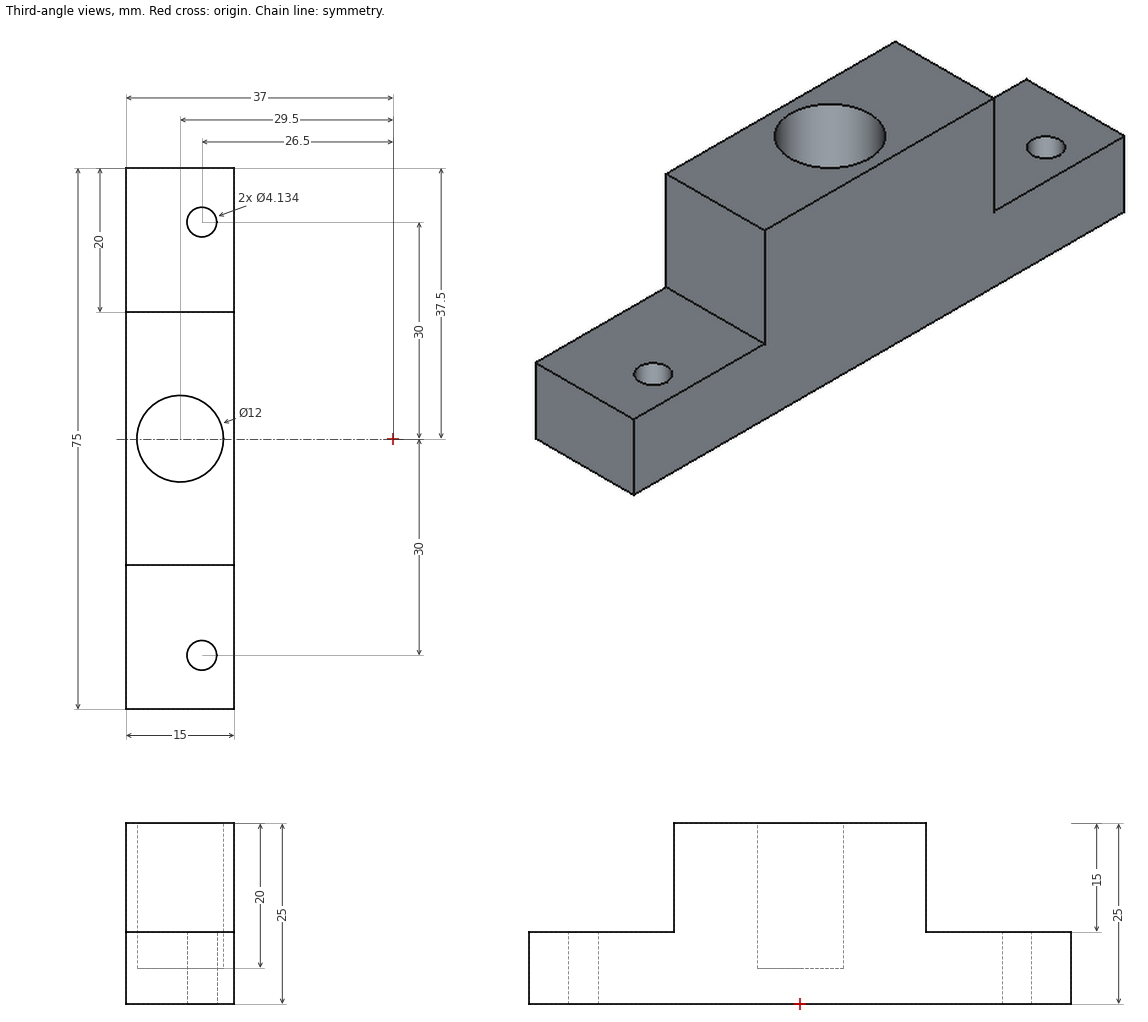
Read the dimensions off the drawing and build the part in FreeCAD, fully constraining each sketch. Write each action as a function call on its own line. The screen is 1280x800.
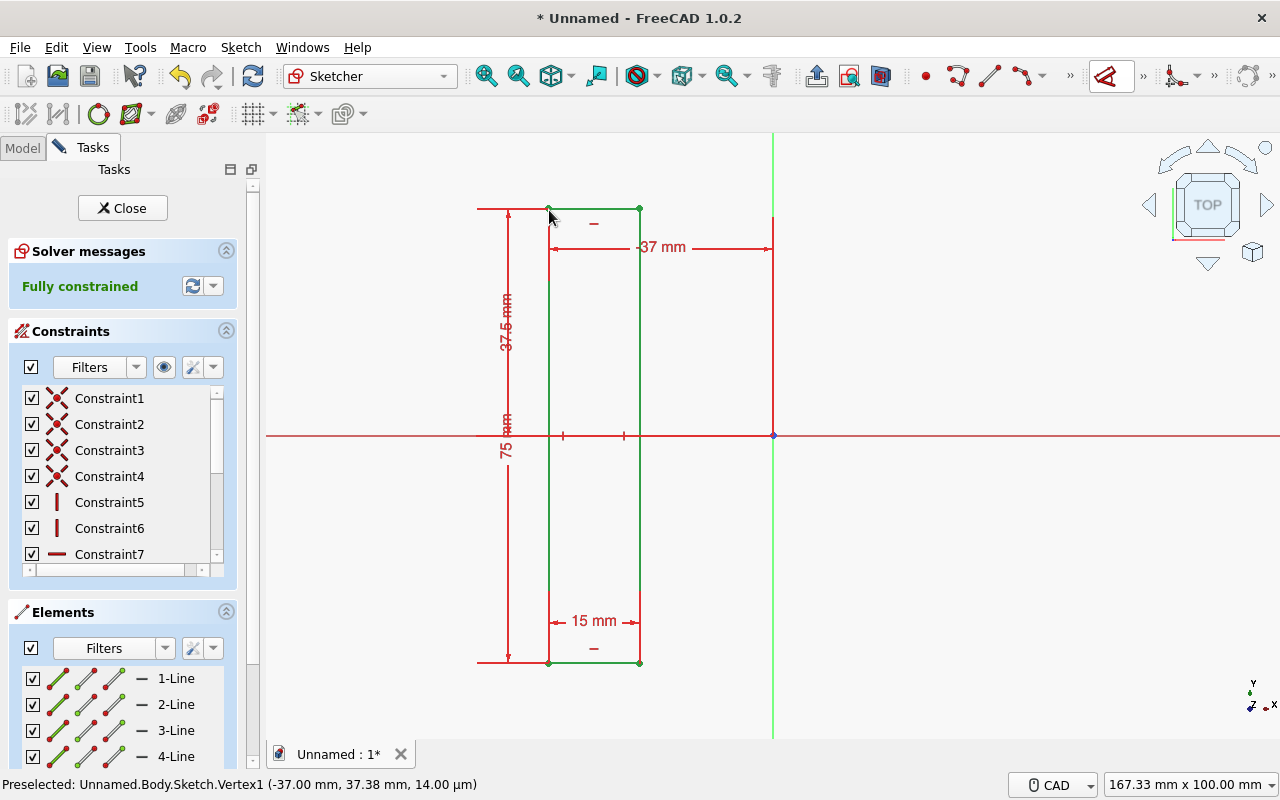
click(123, 208)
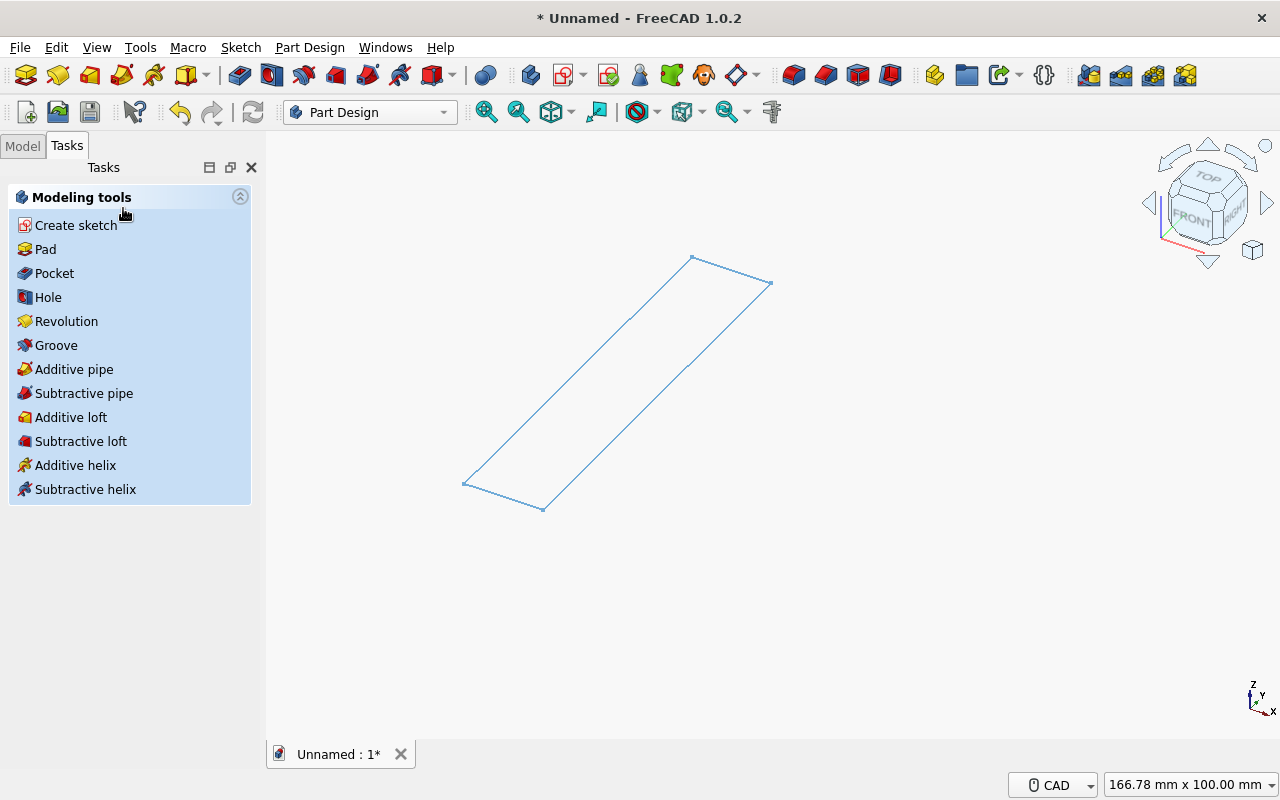
click(26, 76)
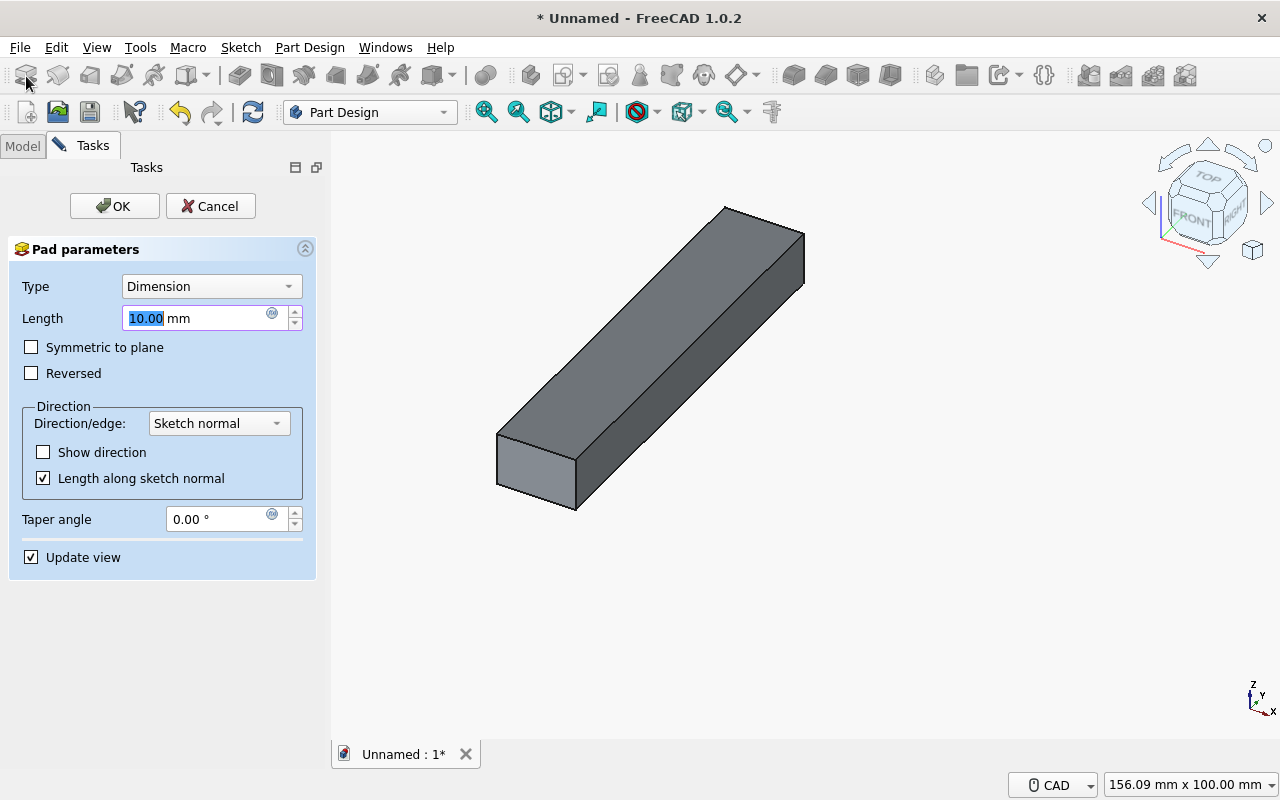
text(25)
key(Tab)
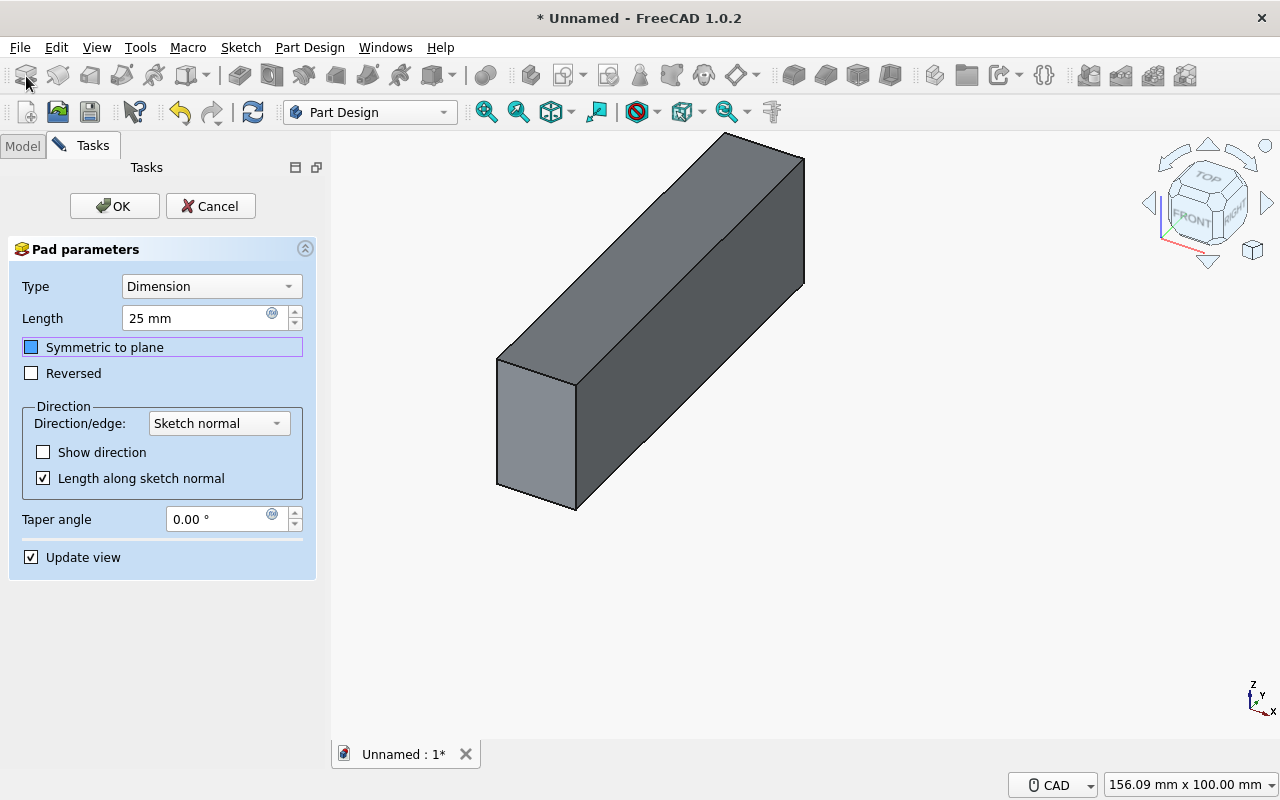
click(115, 206)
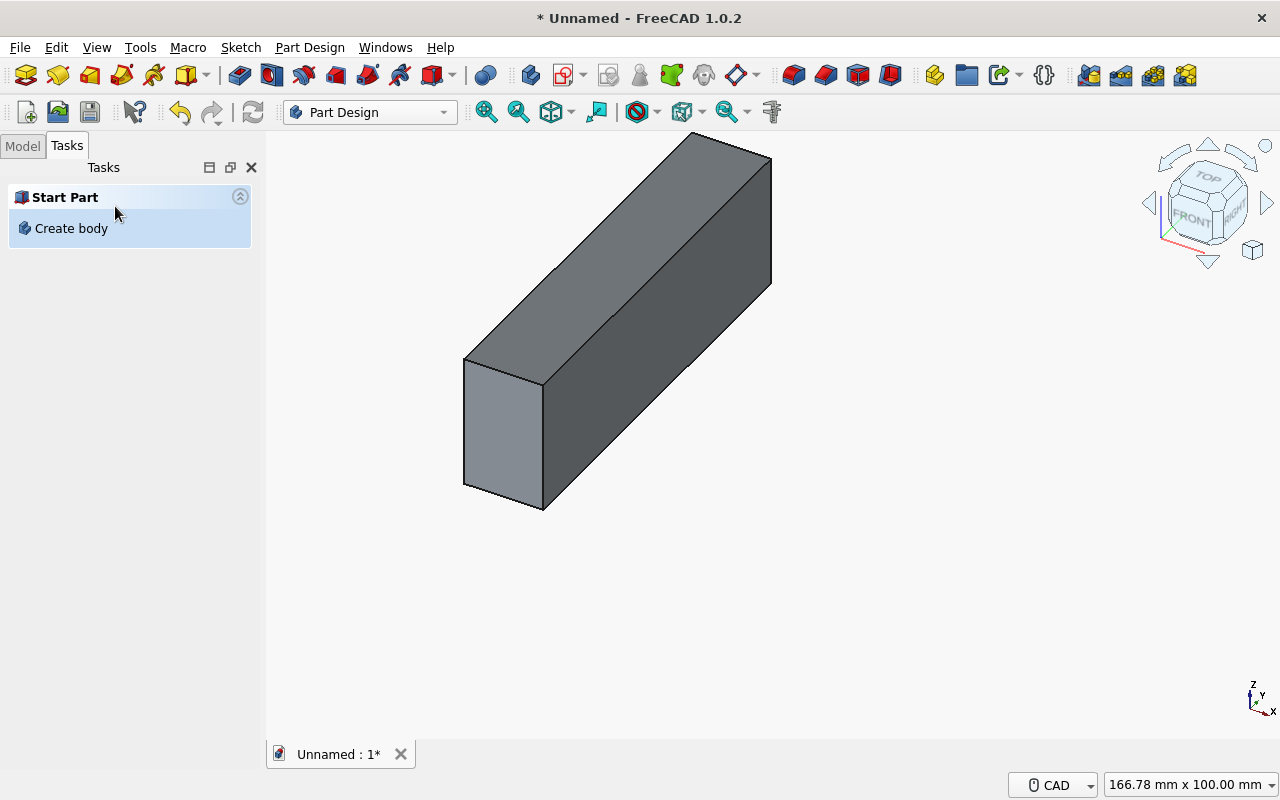
click(683, 193)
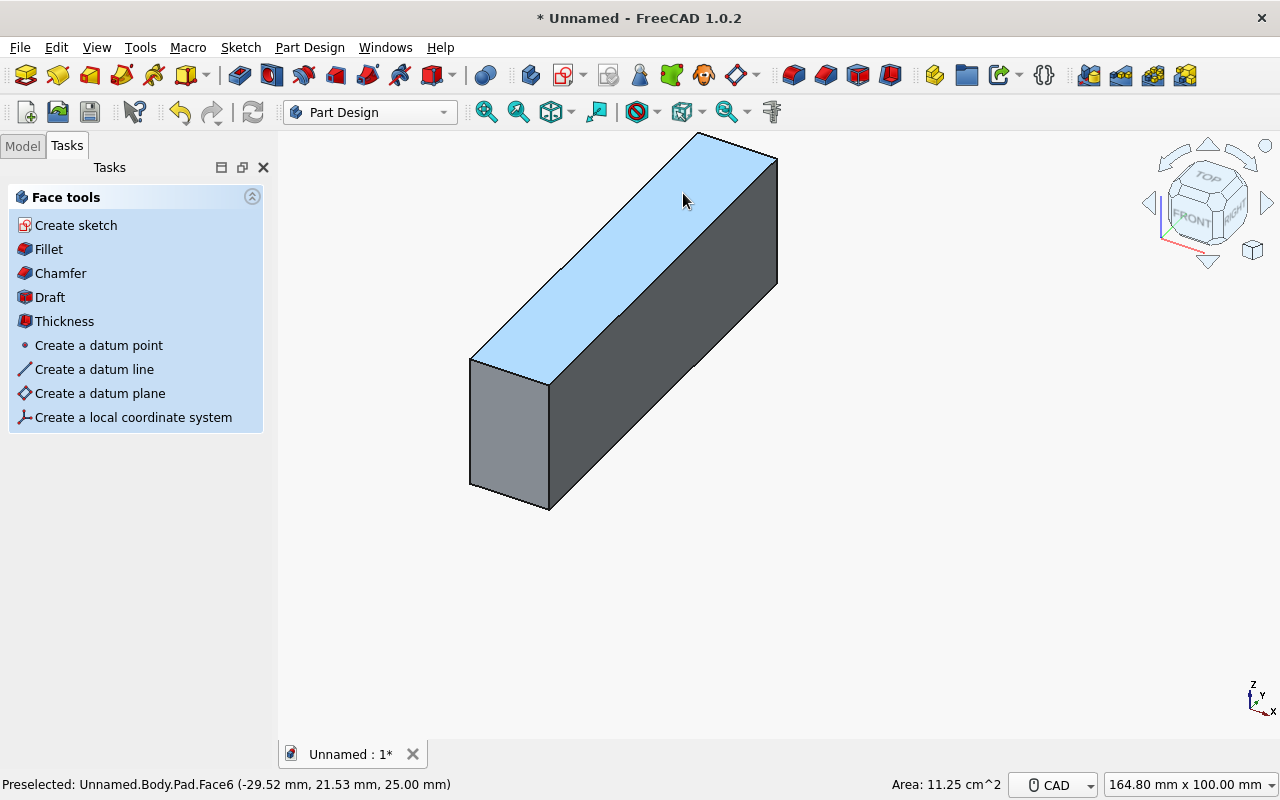
click(564, 76)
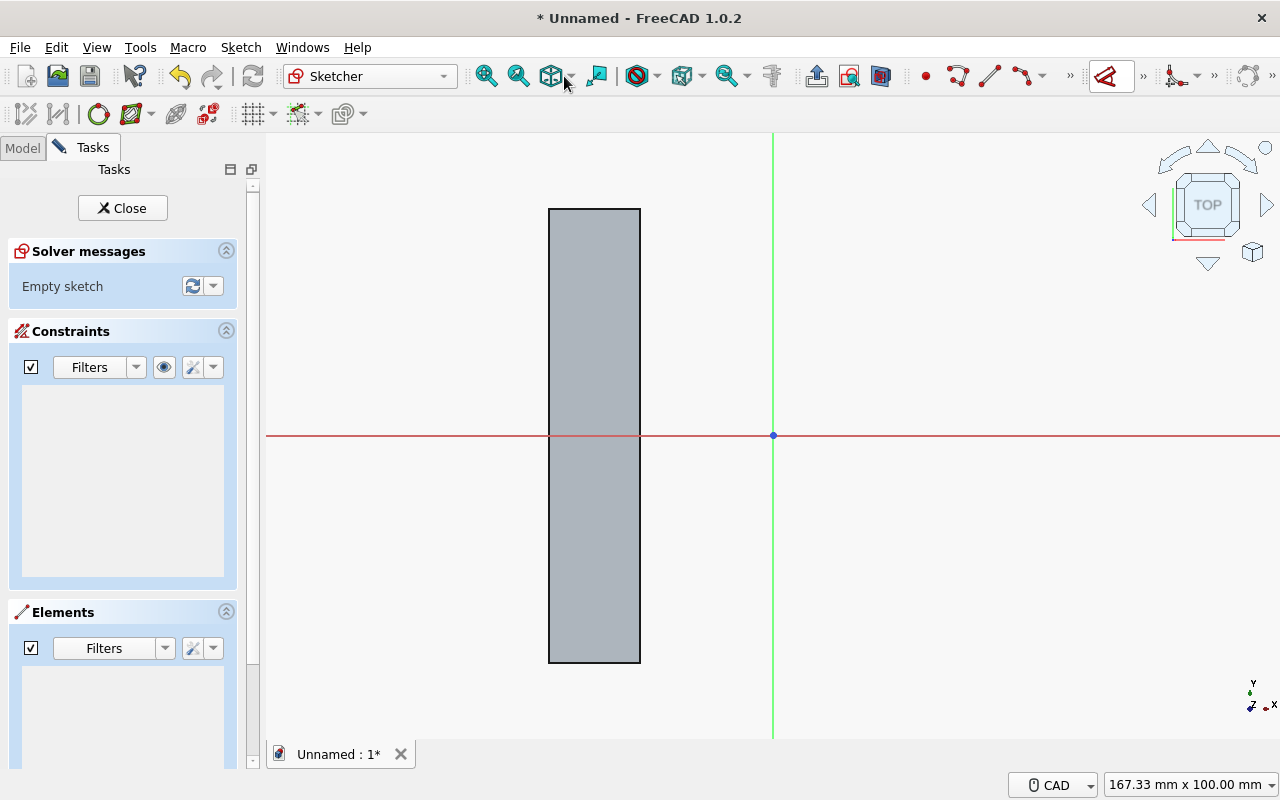
key(g)
key(c)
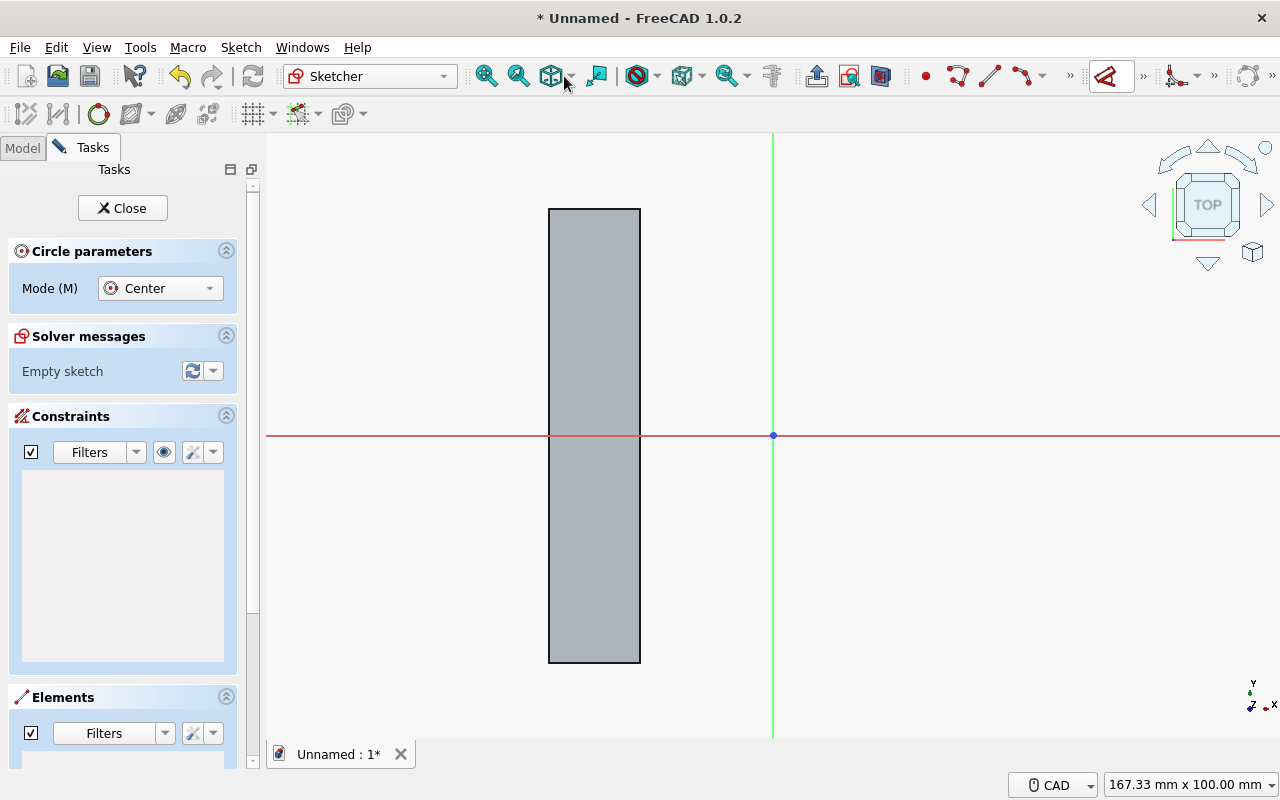
scroll(612, 254, up, 3)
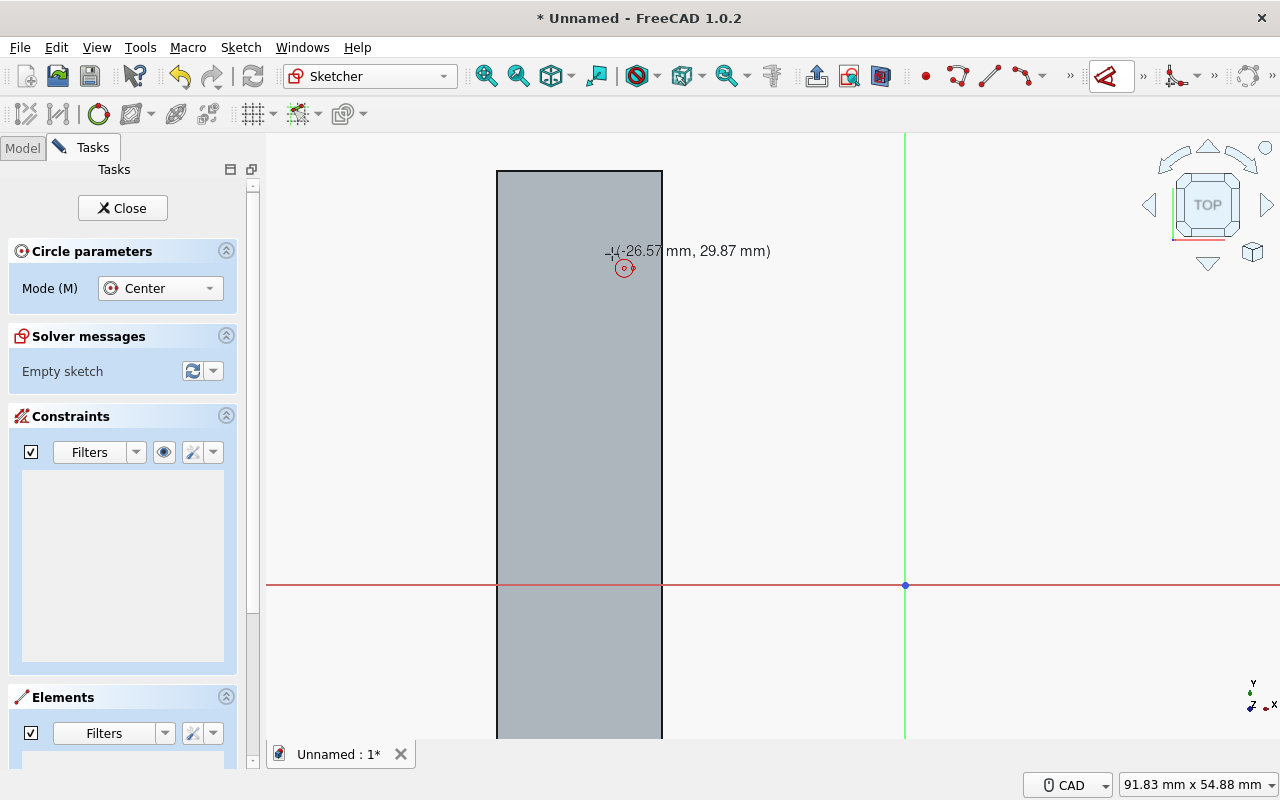
click(612, 254)
click(629, 238)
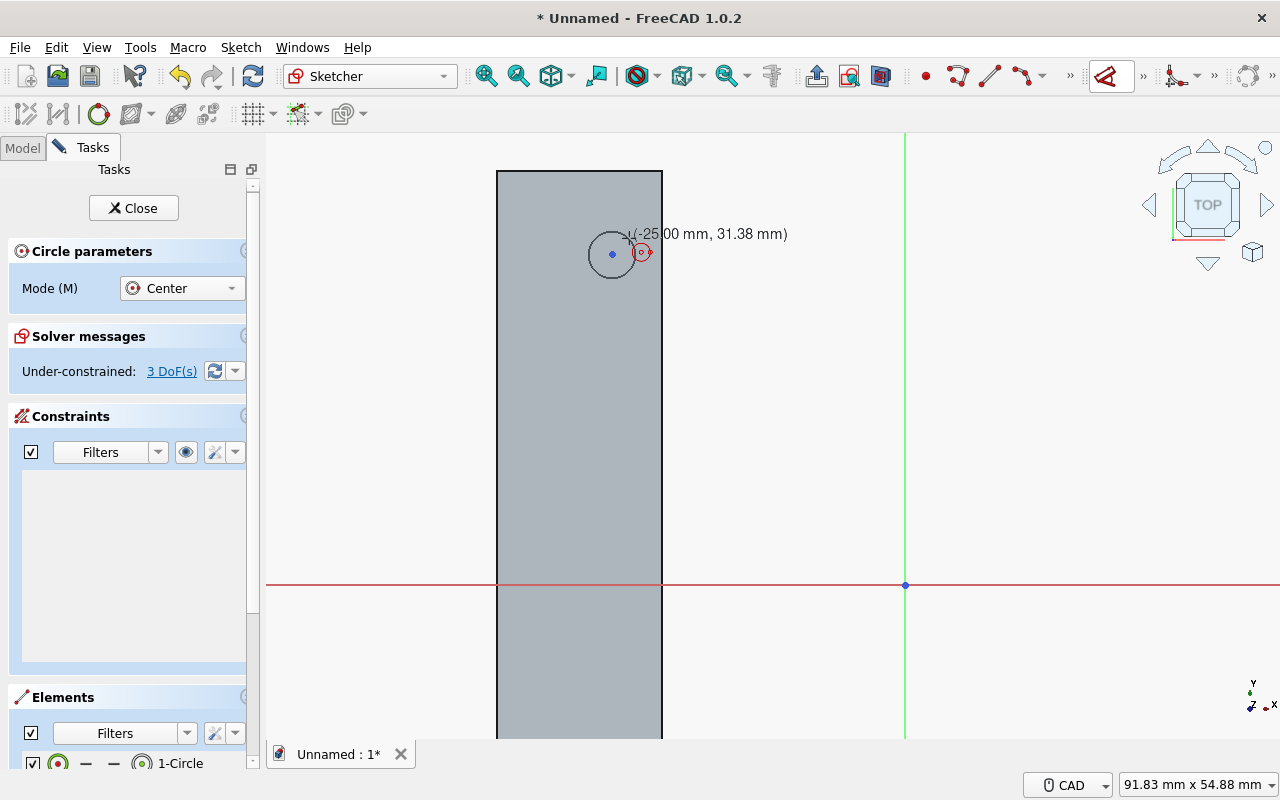
scroll(652, 254, down, 3)